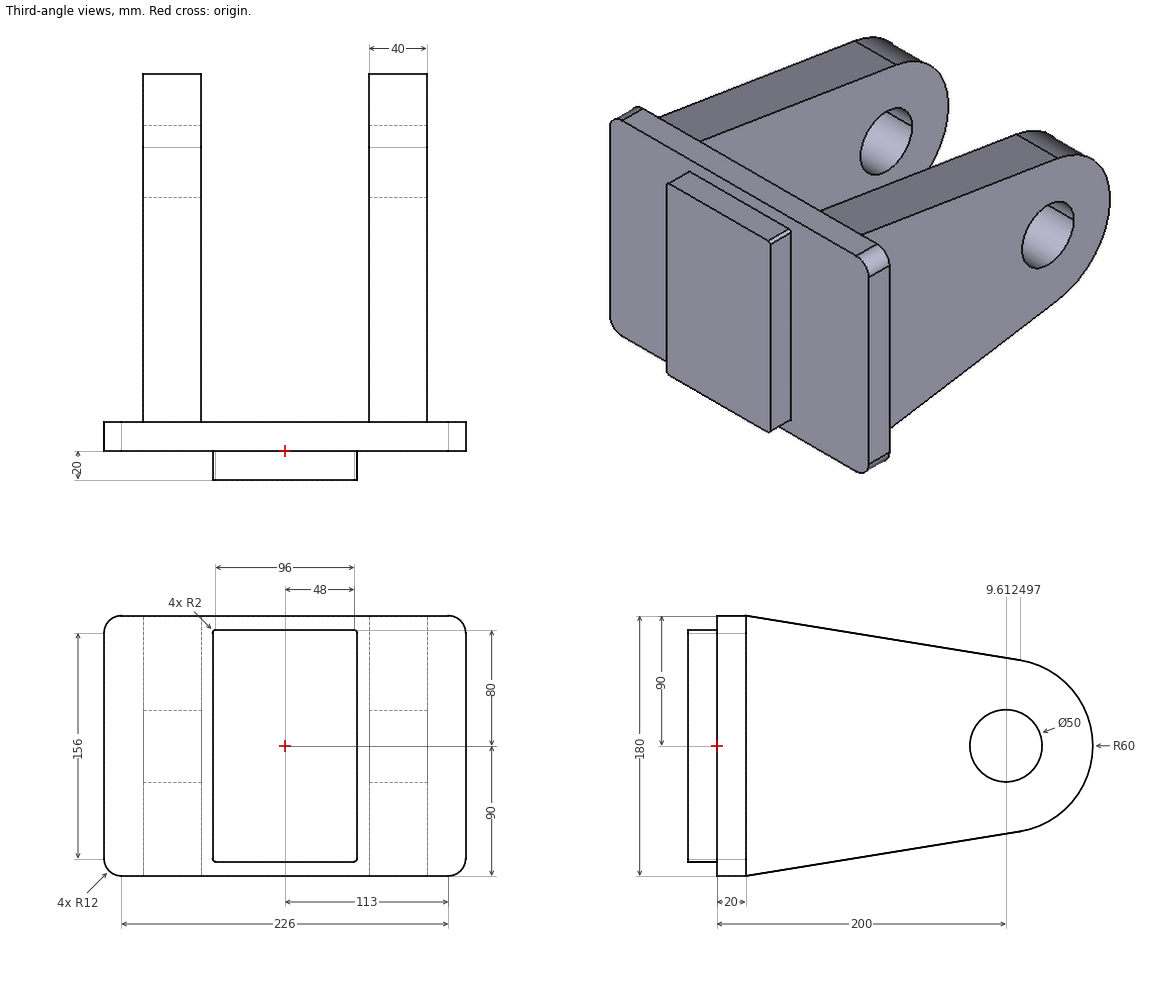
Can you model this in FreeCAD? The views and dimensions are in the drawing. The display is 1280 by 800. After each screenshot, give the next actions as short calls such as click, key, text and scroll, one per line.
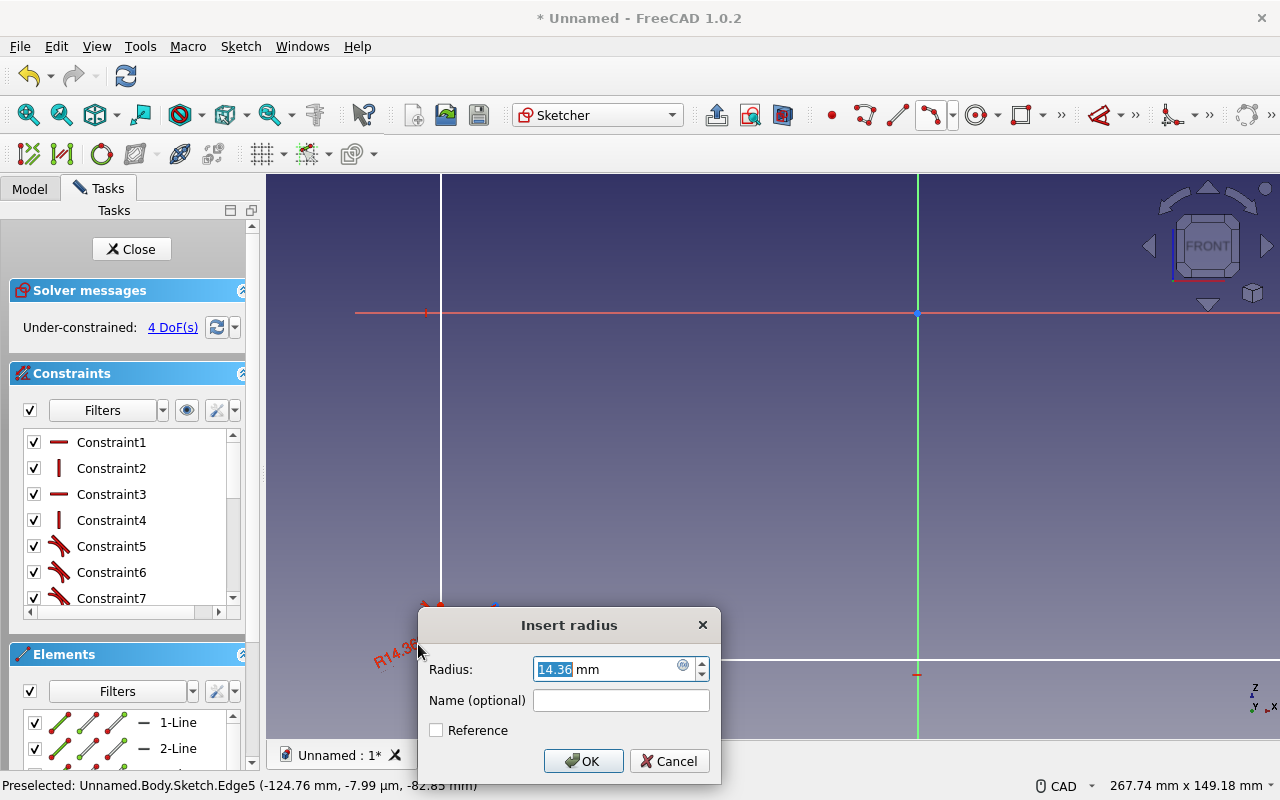
text(12)
key(Return)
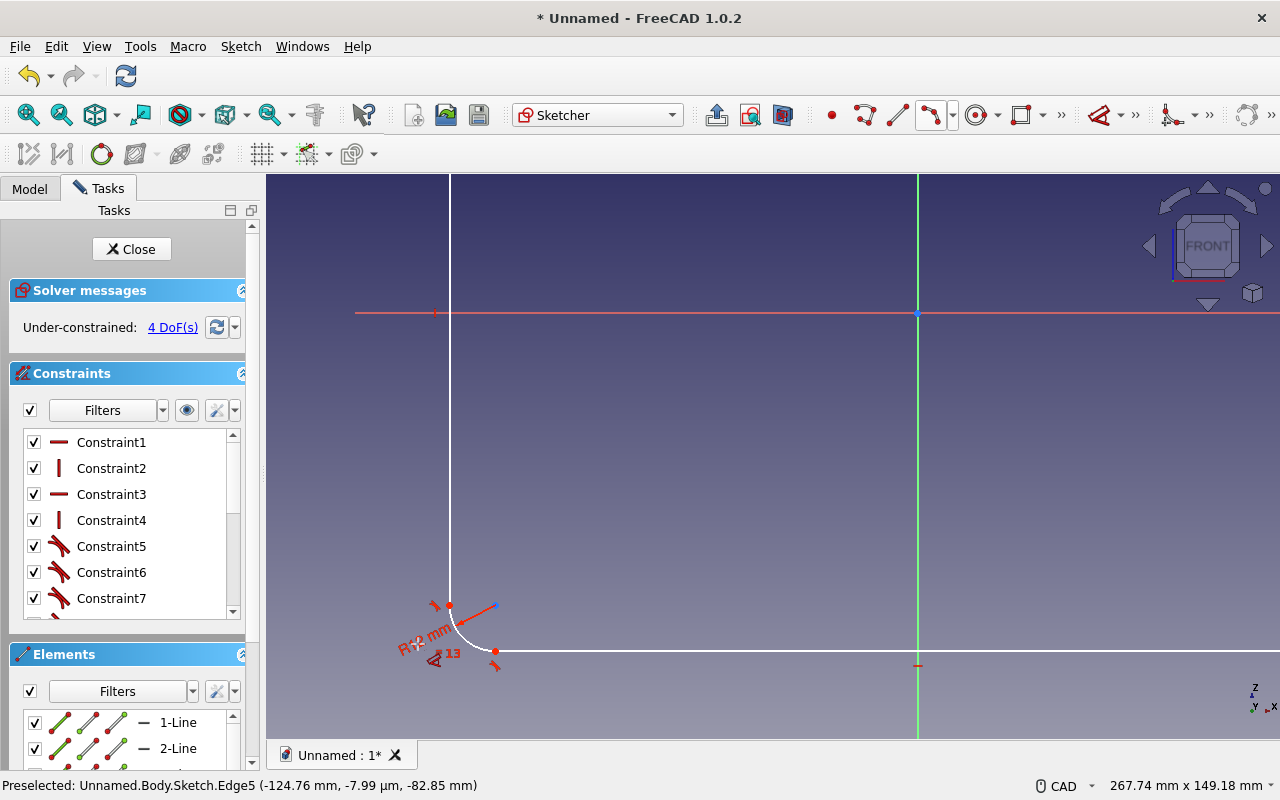
click(1087, 651)
click(805, 685)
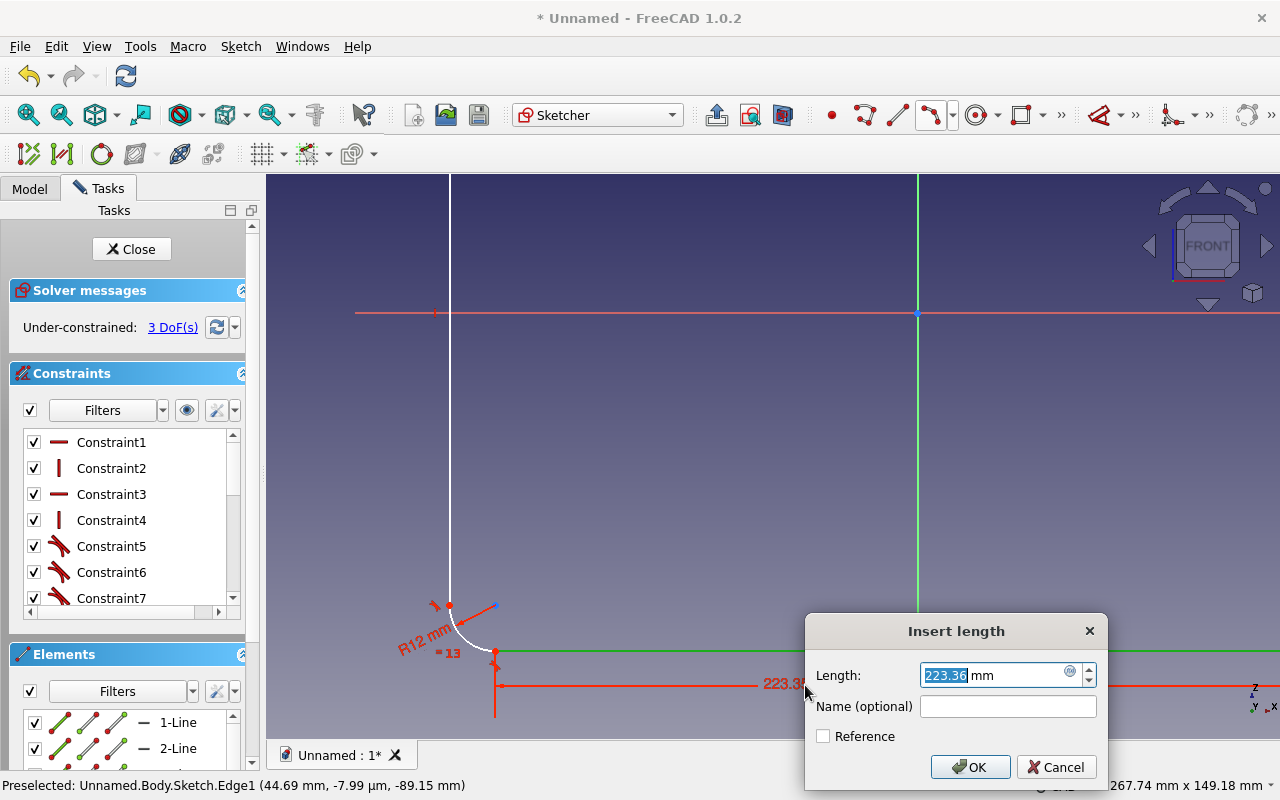
text(226)
key(Return)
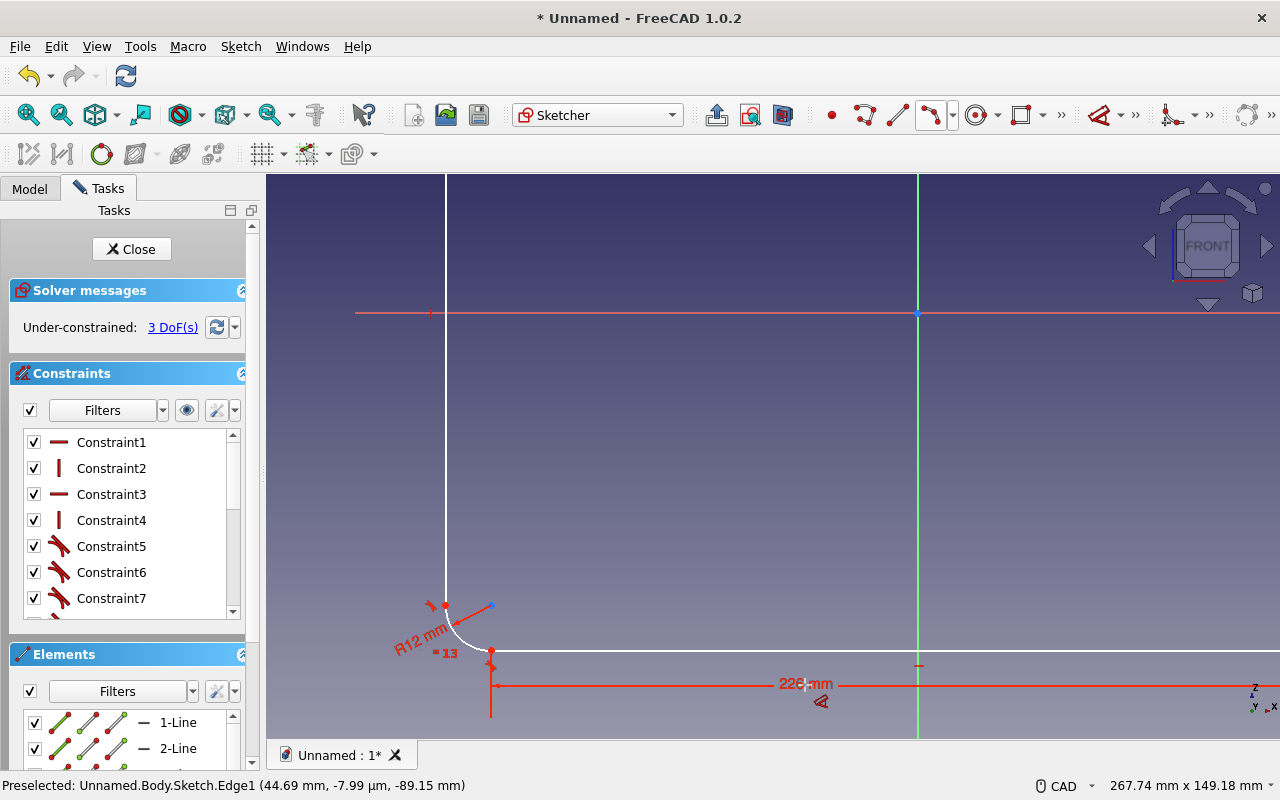
click(446, 430)
click(412, 404)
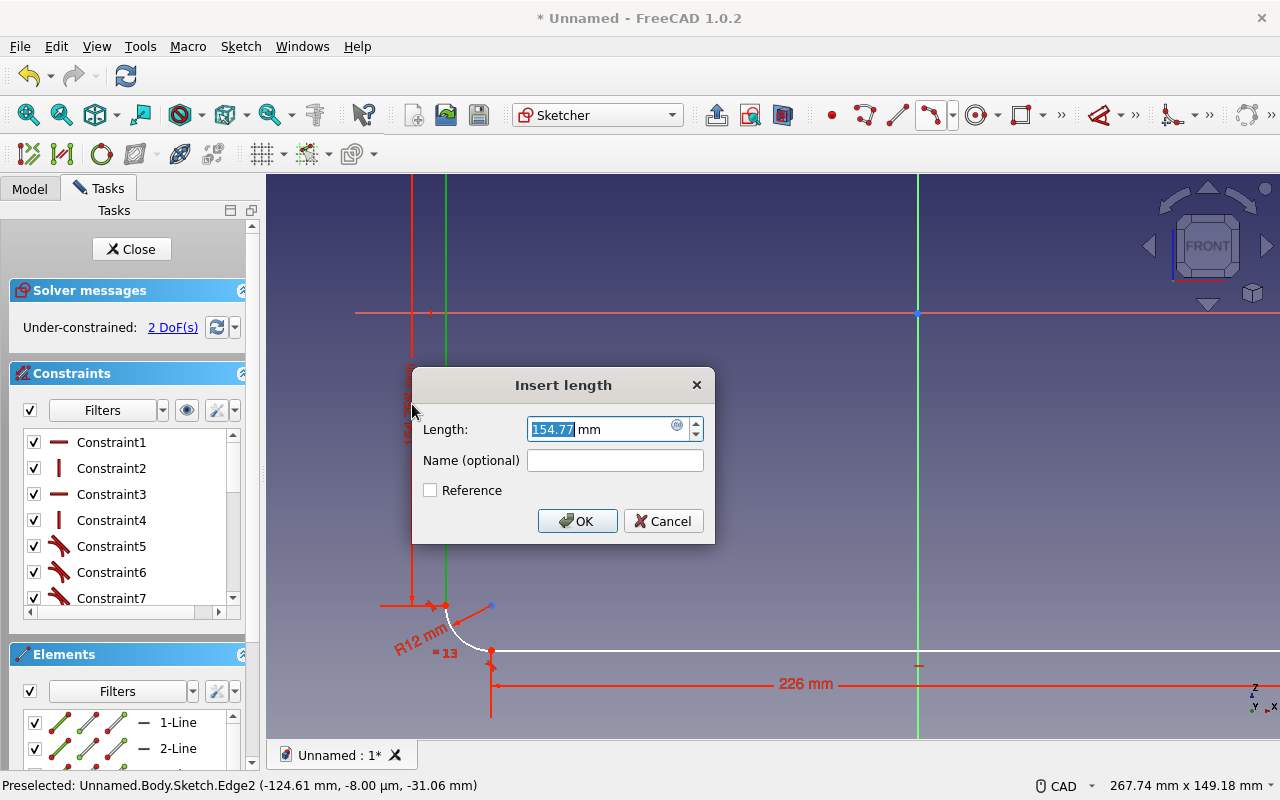
text(156)
key(Return)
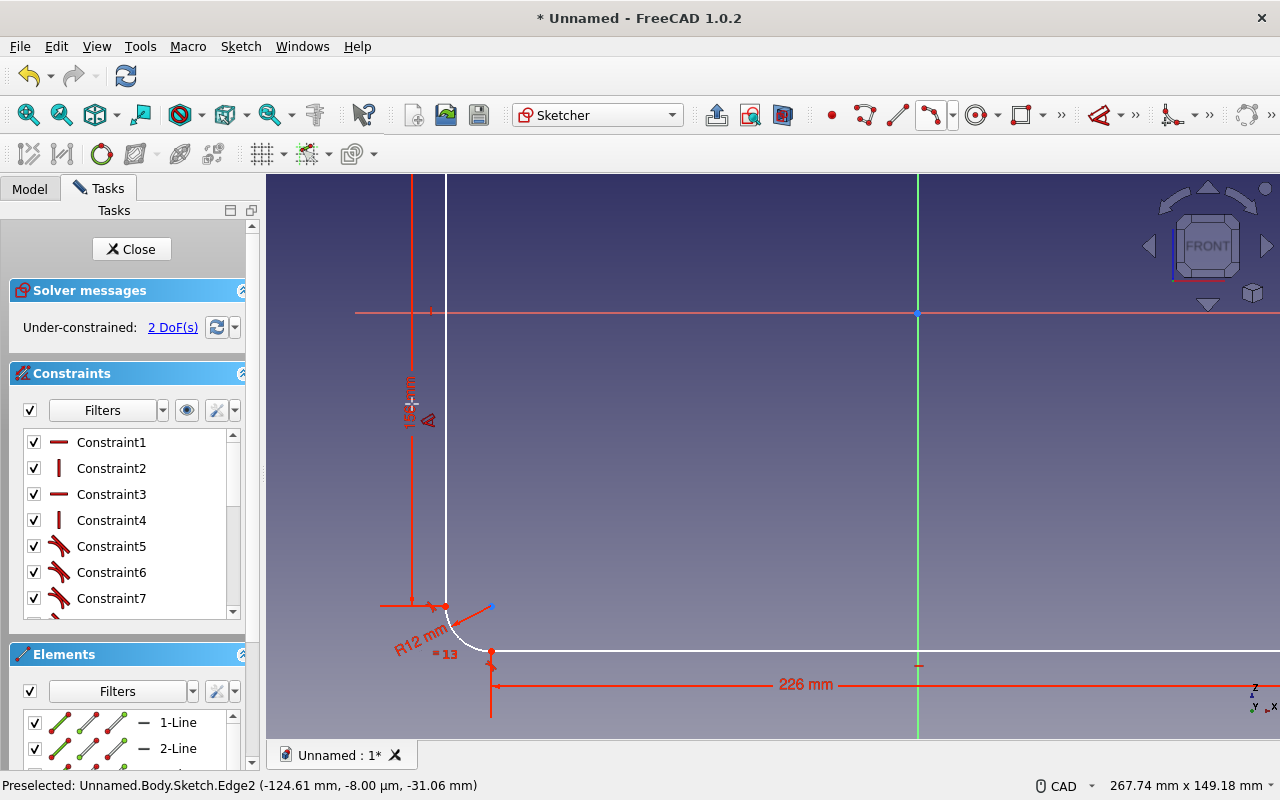
scroll(445, 631, down, 3)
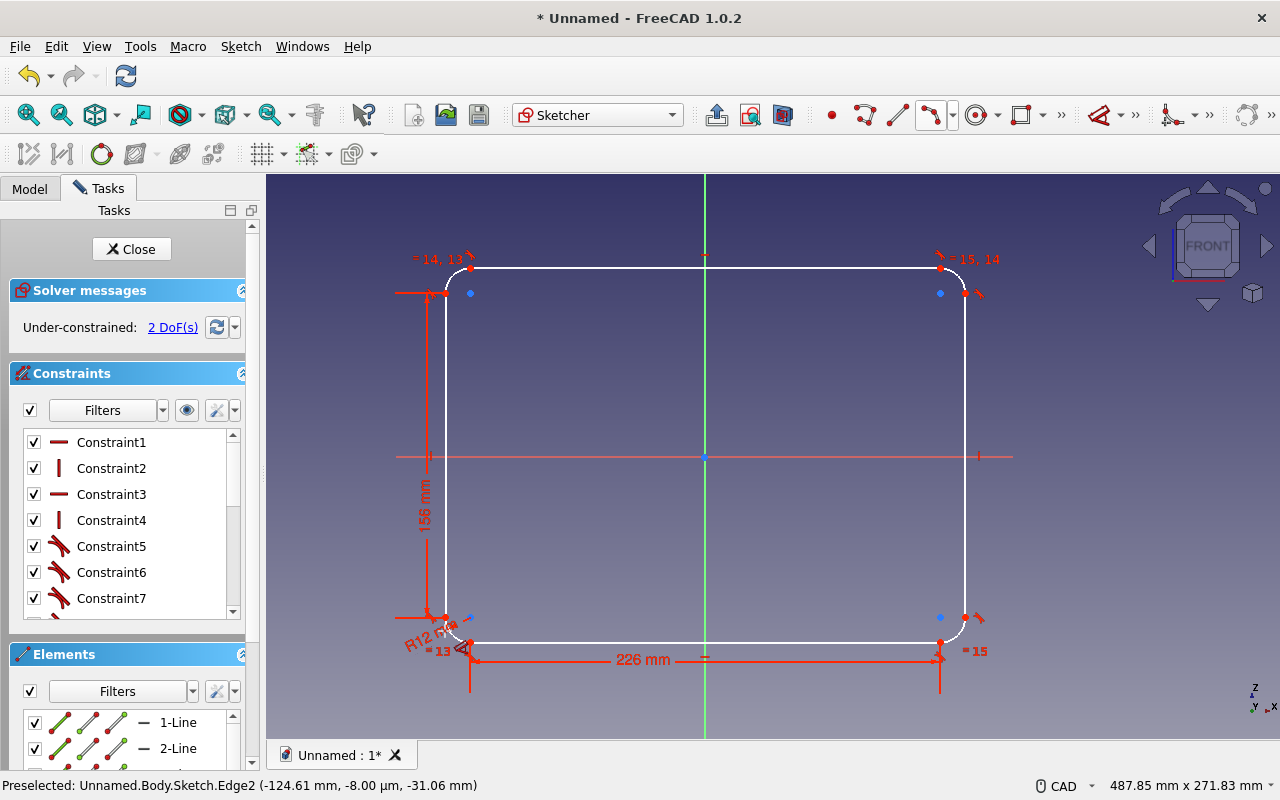
click(940, 643)
click(671, 550)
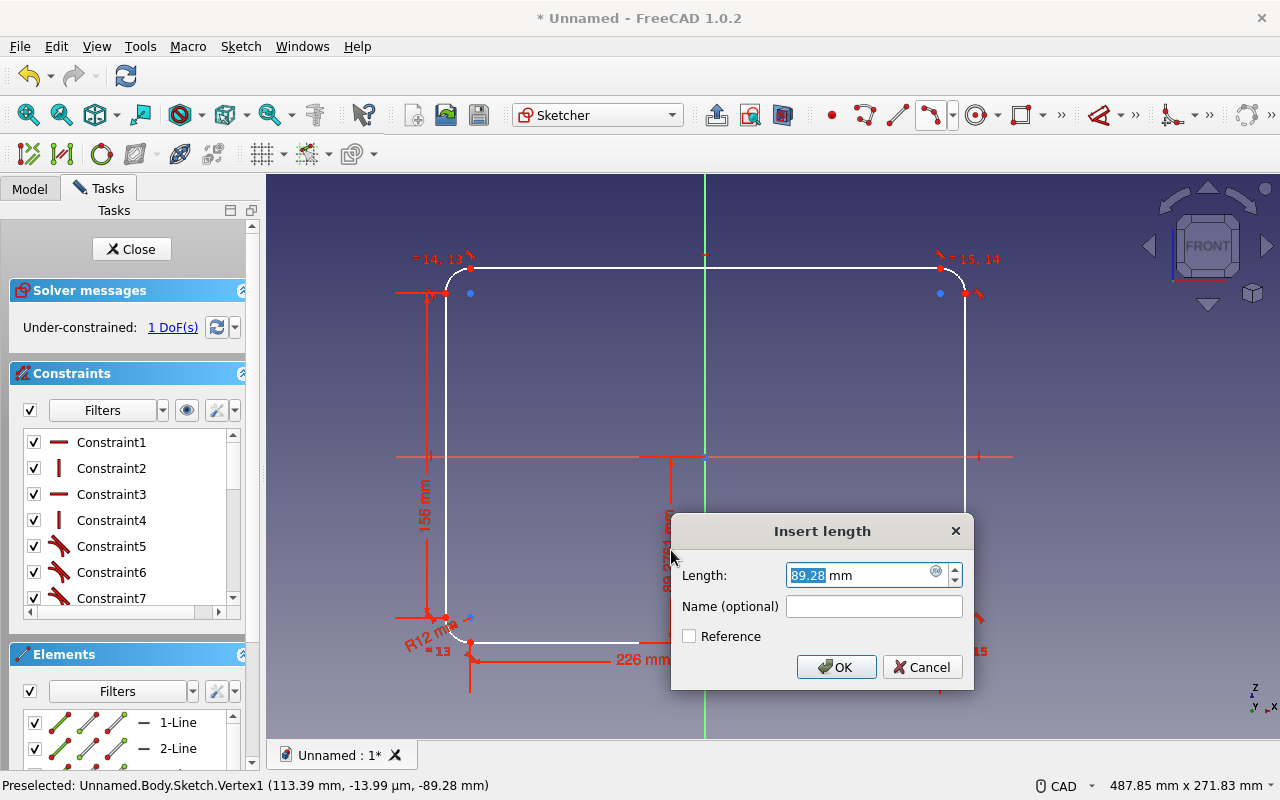
text(90)
key(Return)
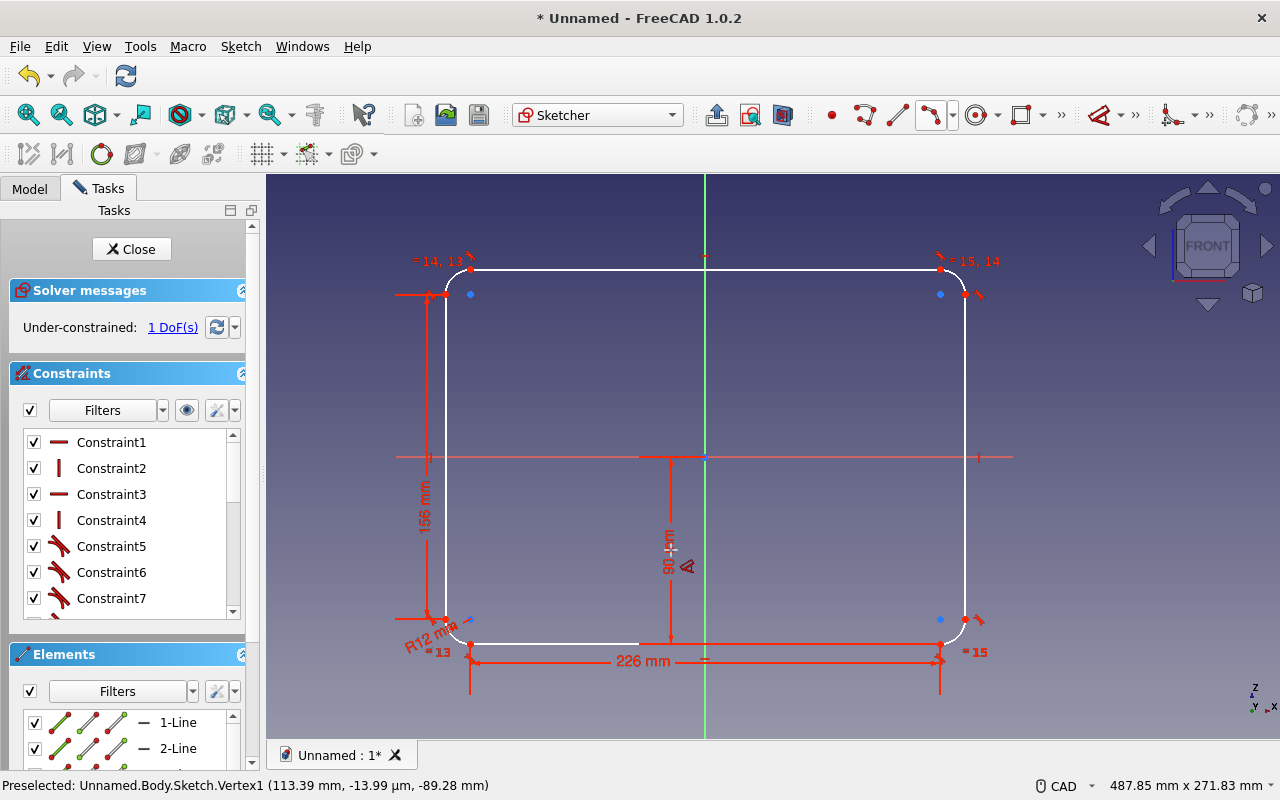
click(940, 644)
click(822, 678)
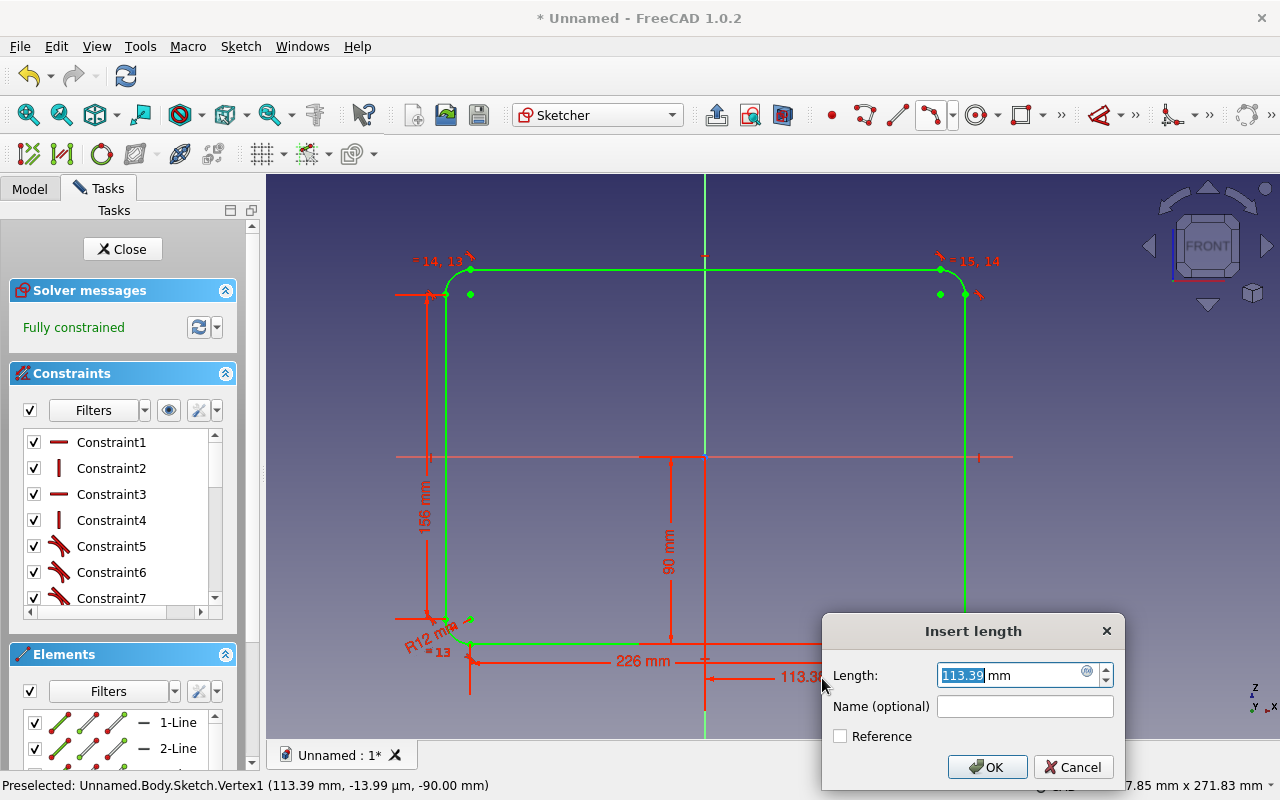
text(113)
key(Return)
key(Escape)